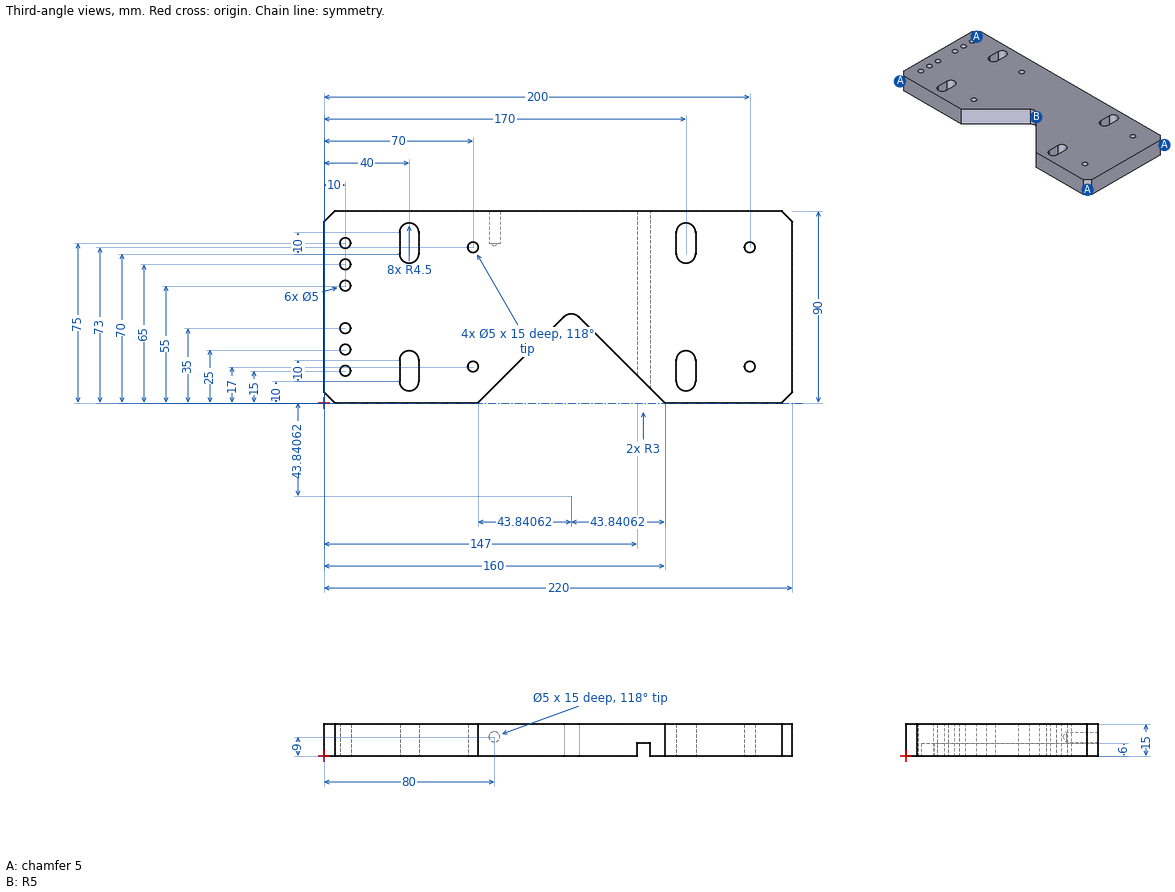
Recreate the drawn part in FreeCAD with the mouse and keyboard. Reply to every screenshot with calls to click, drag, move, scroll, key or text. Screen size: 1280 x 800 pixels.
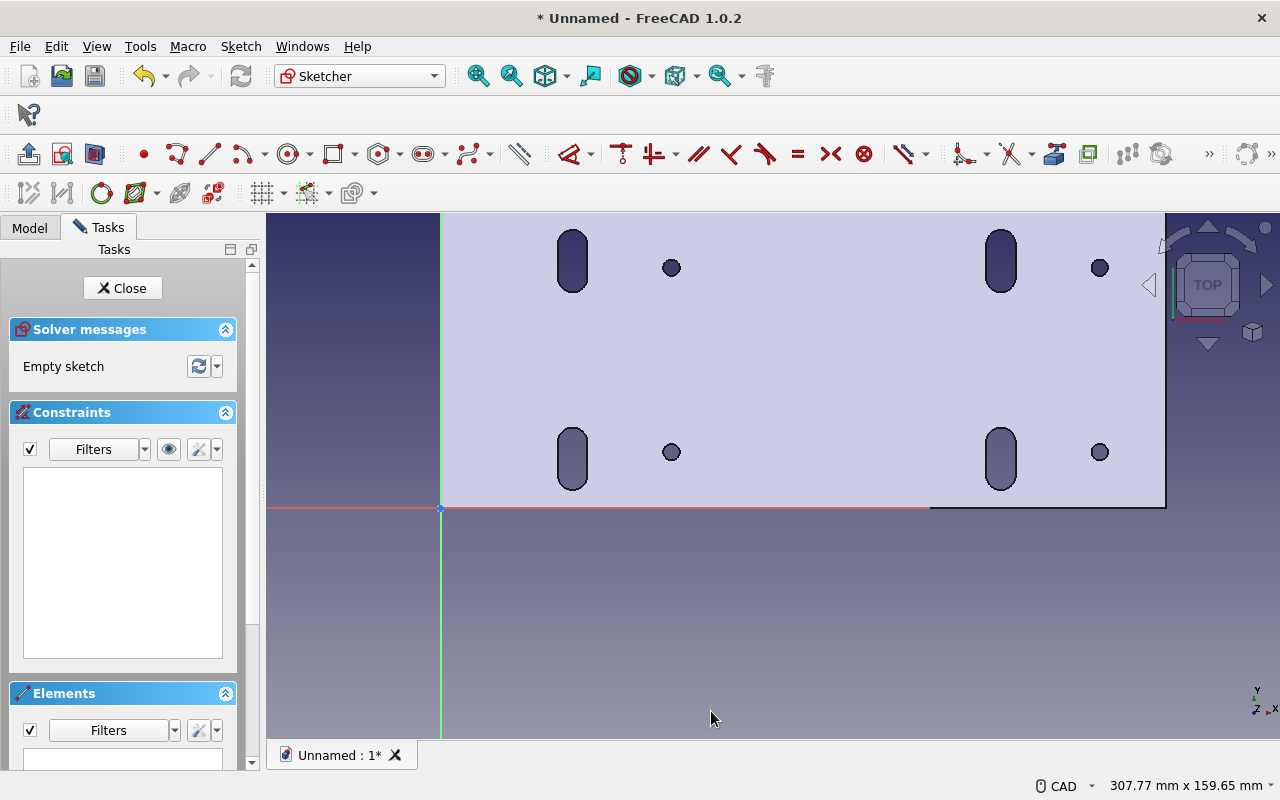
key(g)
key(m)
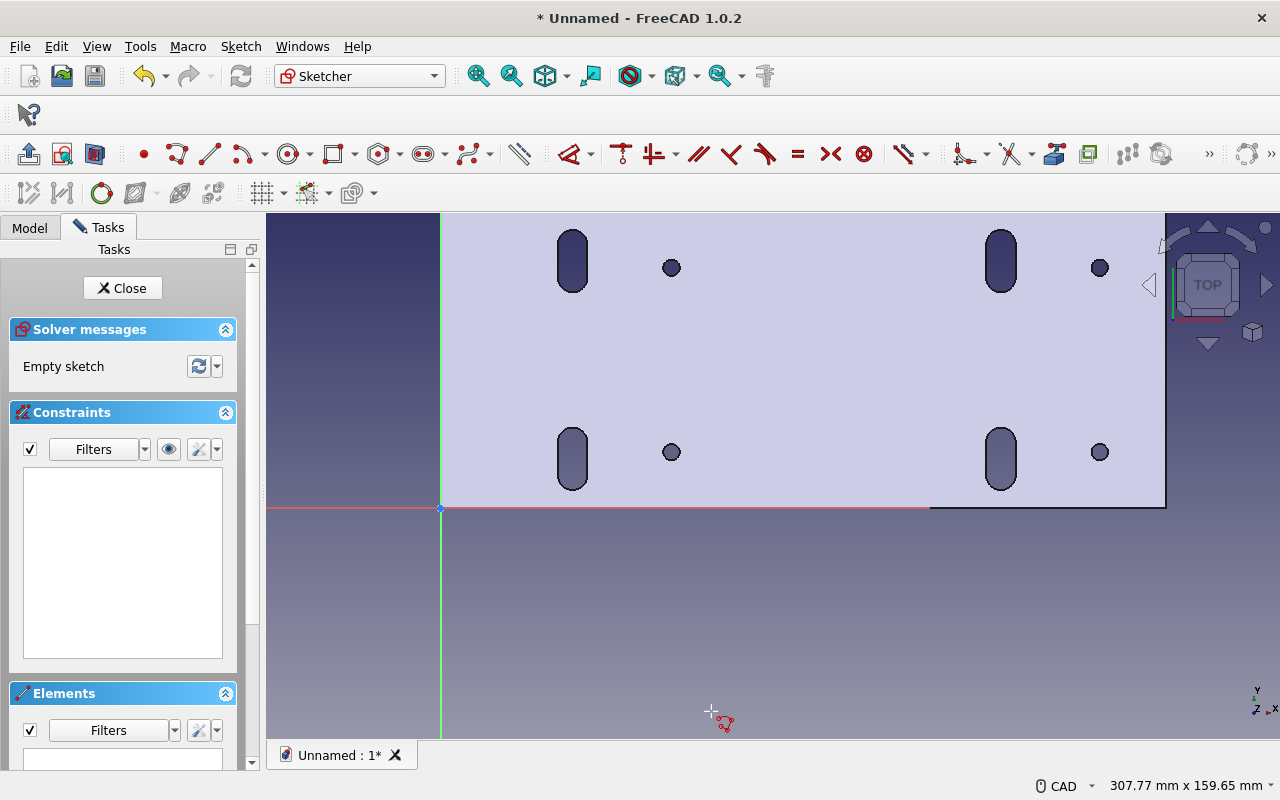
click(679, 508)
click(824, 653)
click(968, 508)
click(824, 364)
click(679, 508)
key(Escape)
key(Escape)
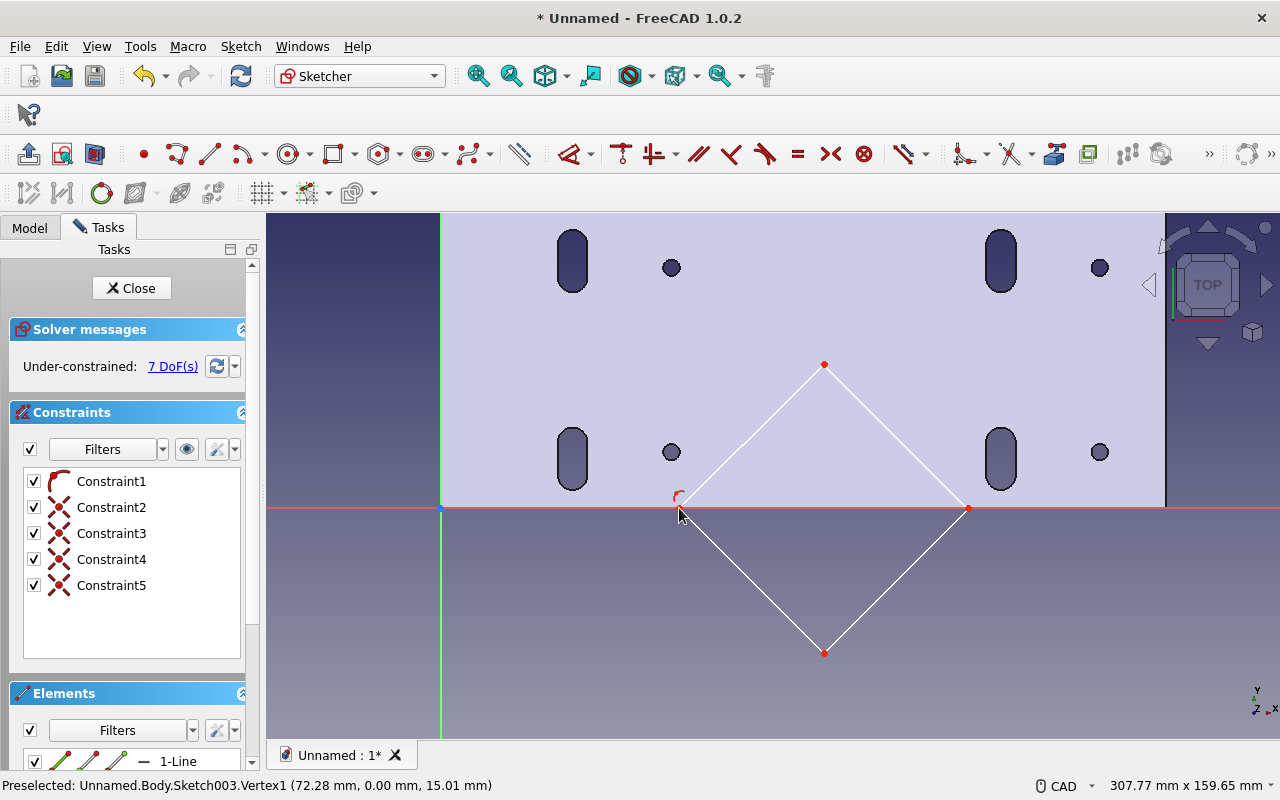
click(824, 654)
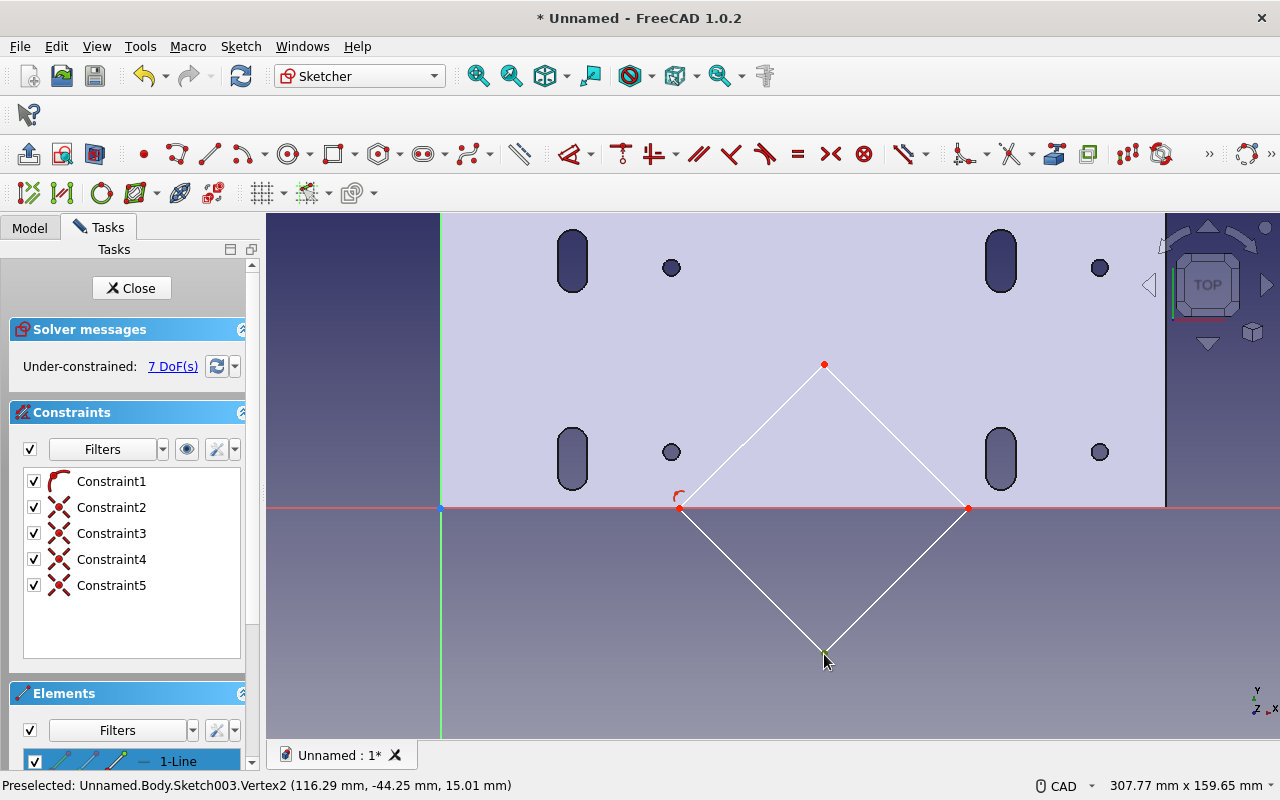
click(824, 365)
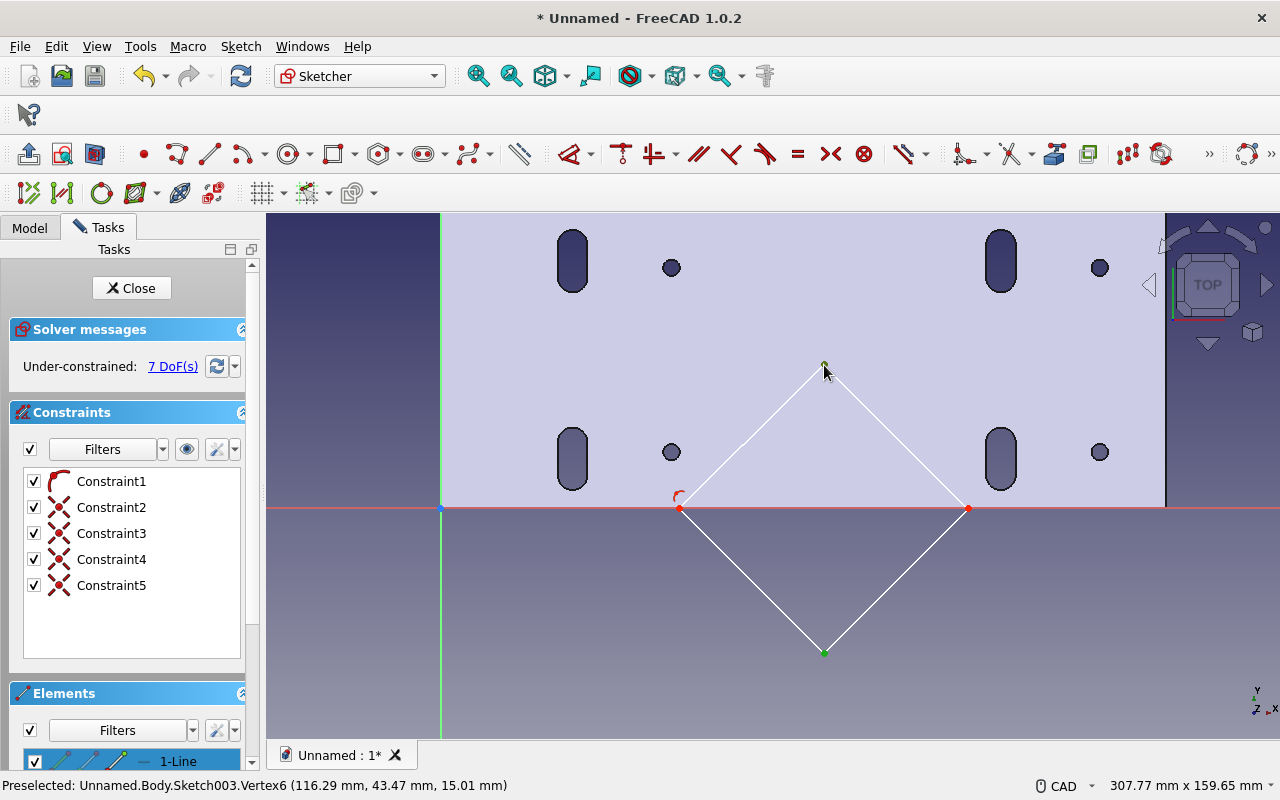
click(353, 508)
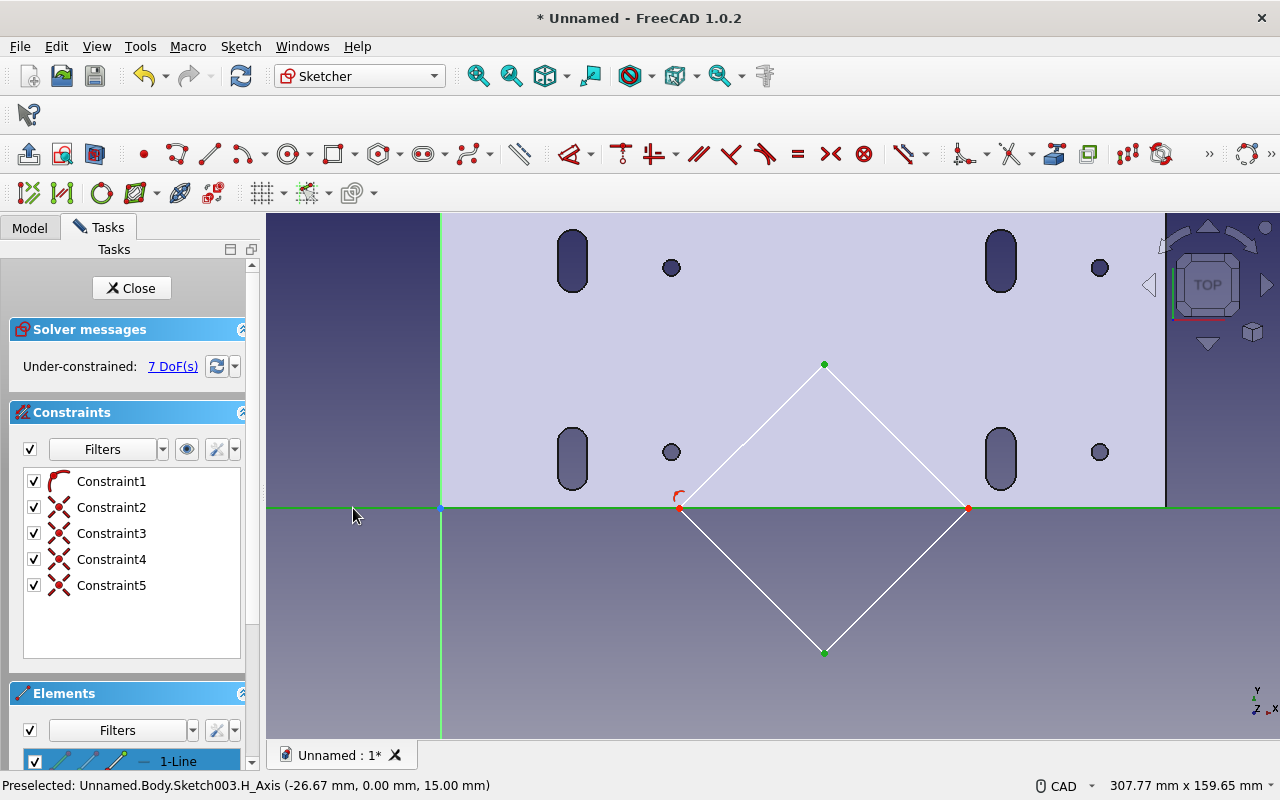
key(s)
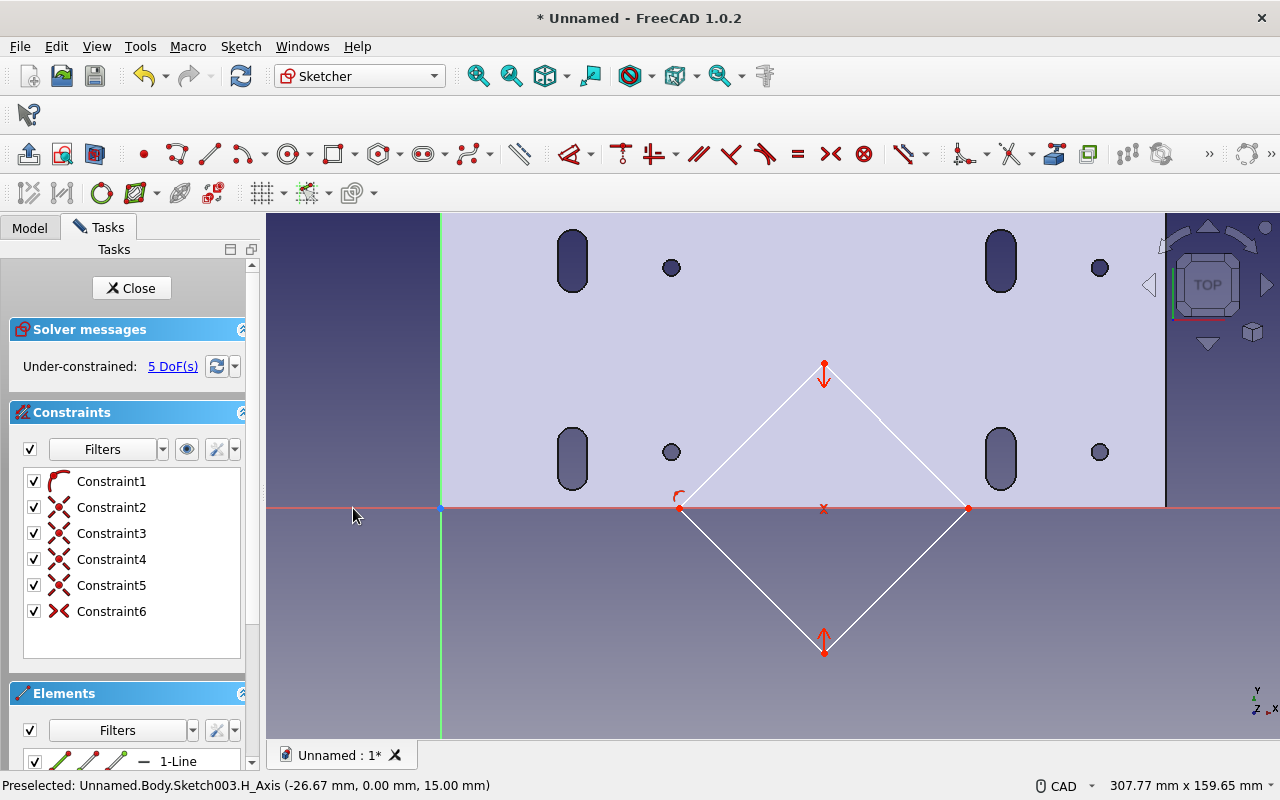
click(968, 509)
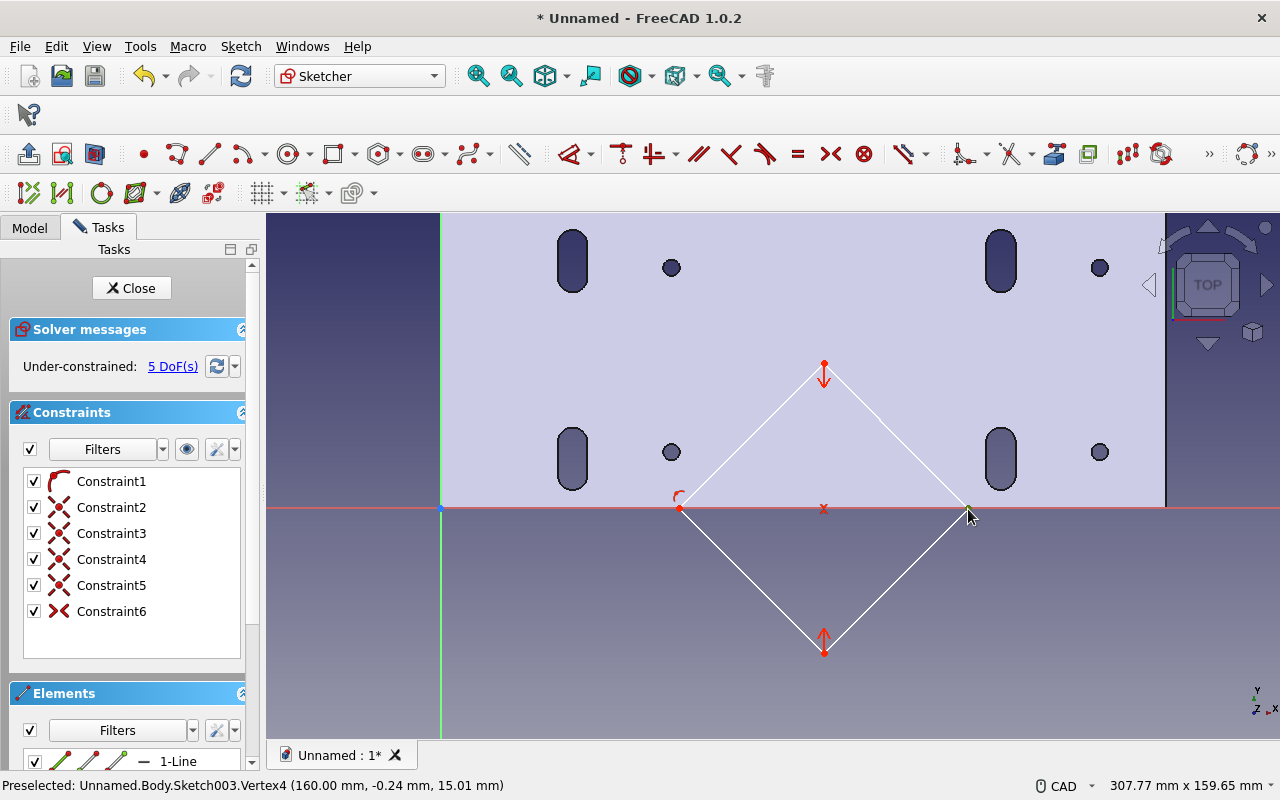
click(353, 508)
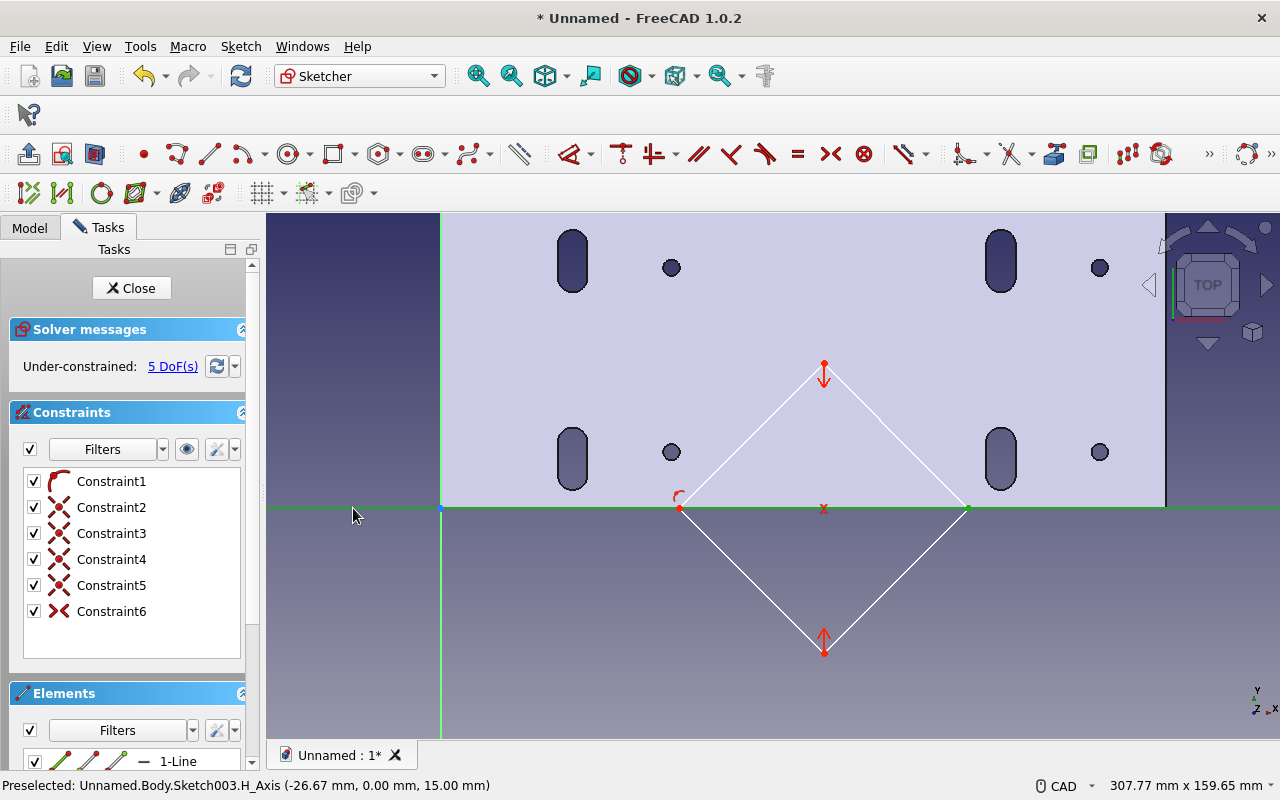
key(c)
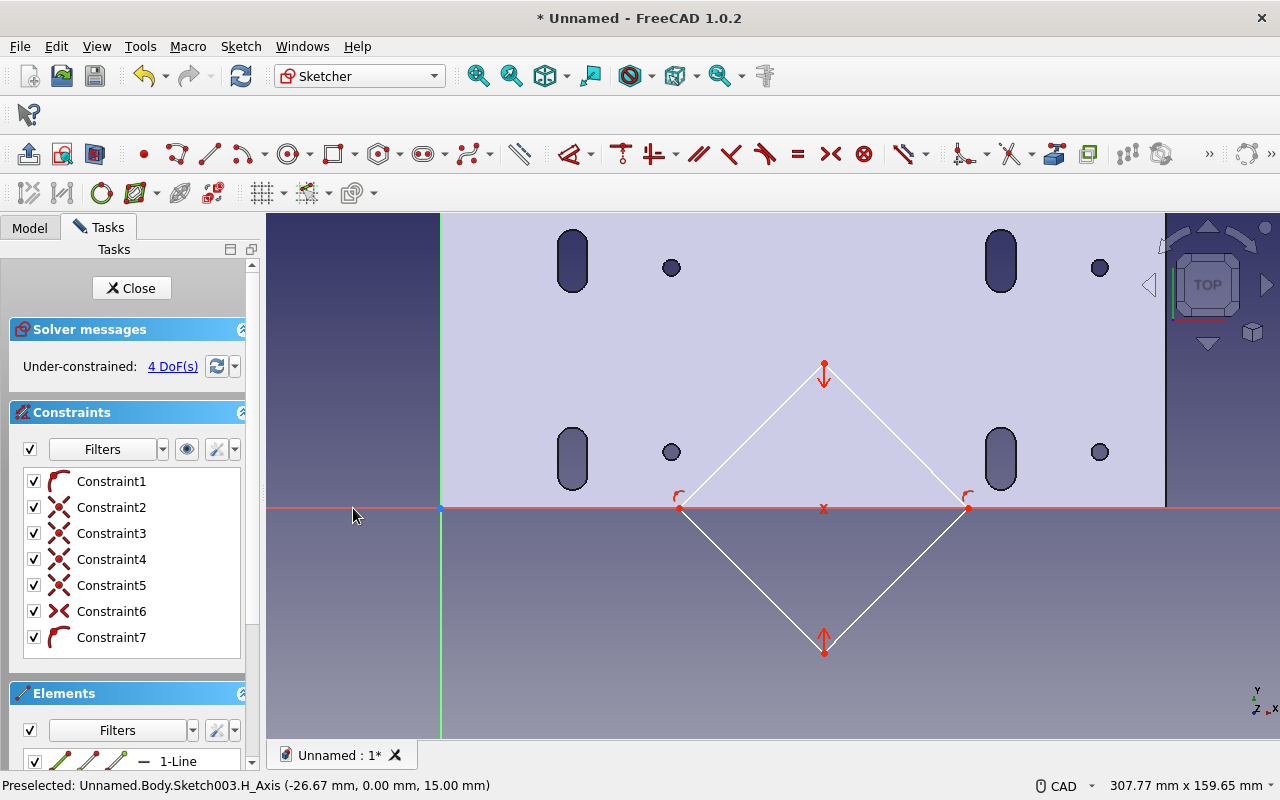
key(d)